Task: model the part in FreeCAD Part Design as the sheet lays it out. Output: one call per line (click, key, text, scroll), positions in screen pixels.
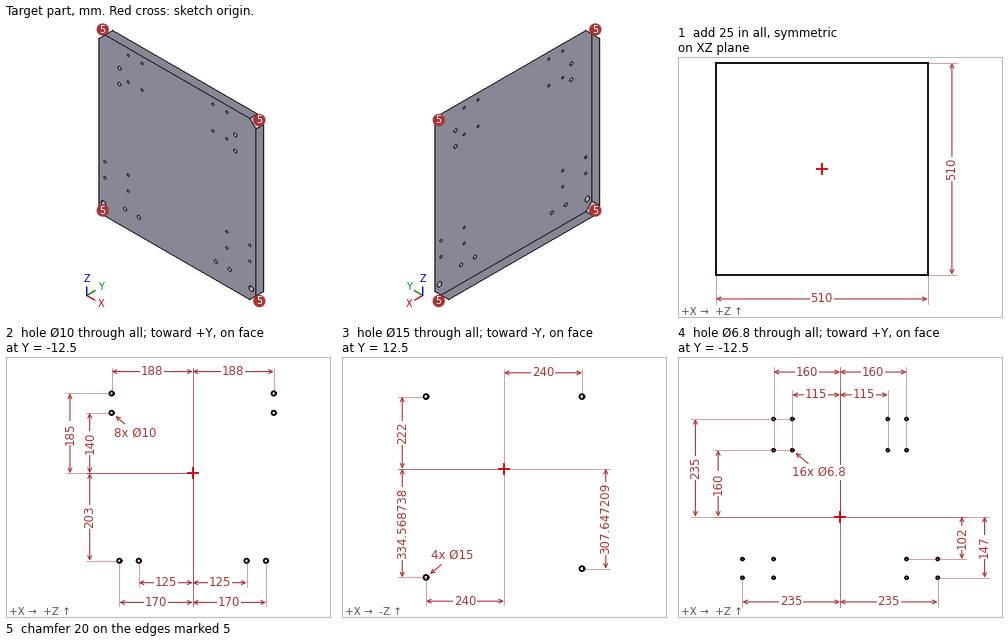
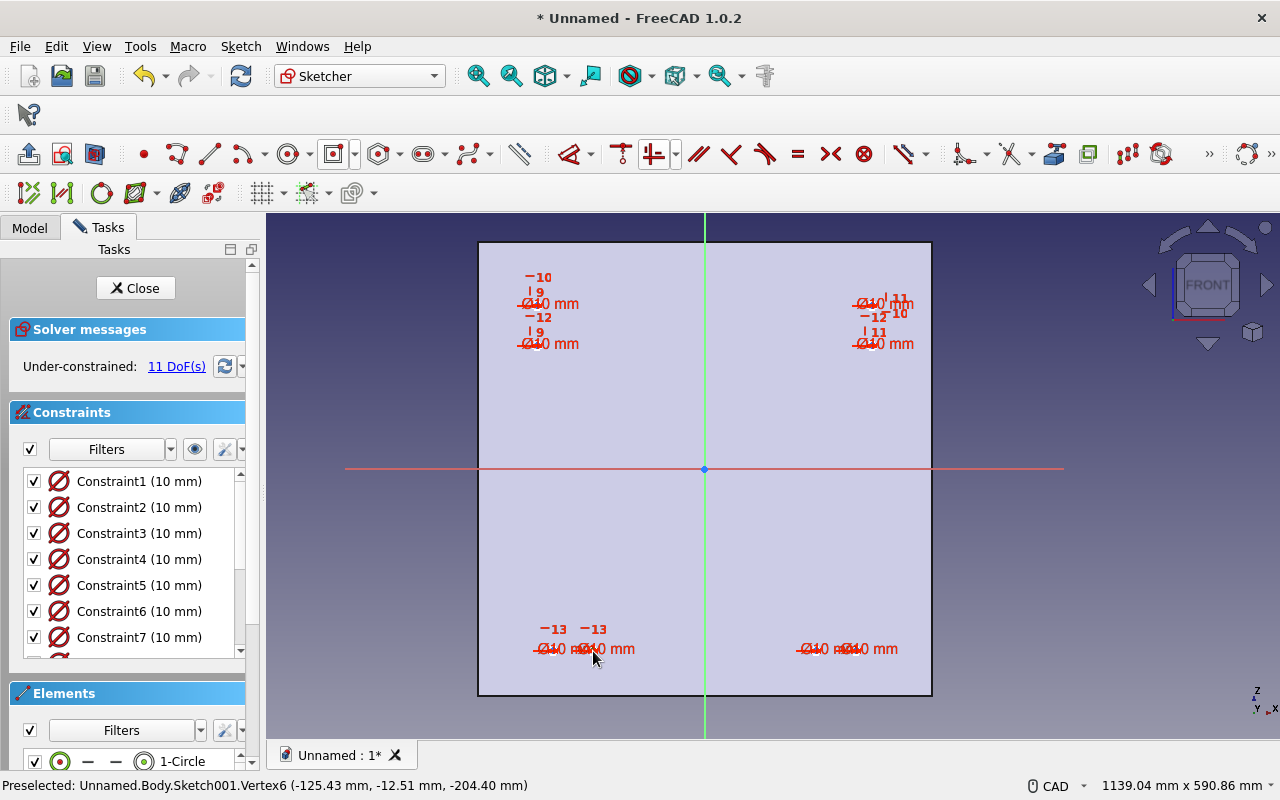
click(816, 651)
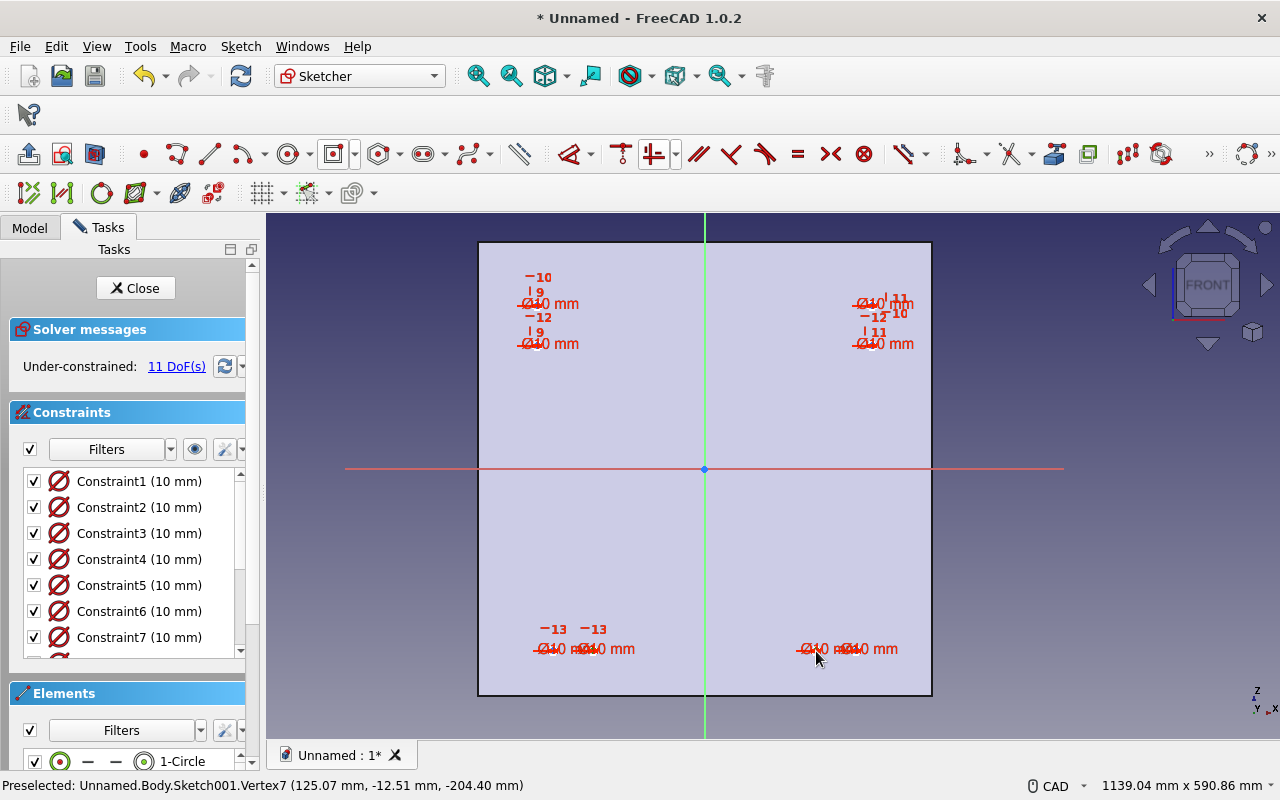
click(676, 154)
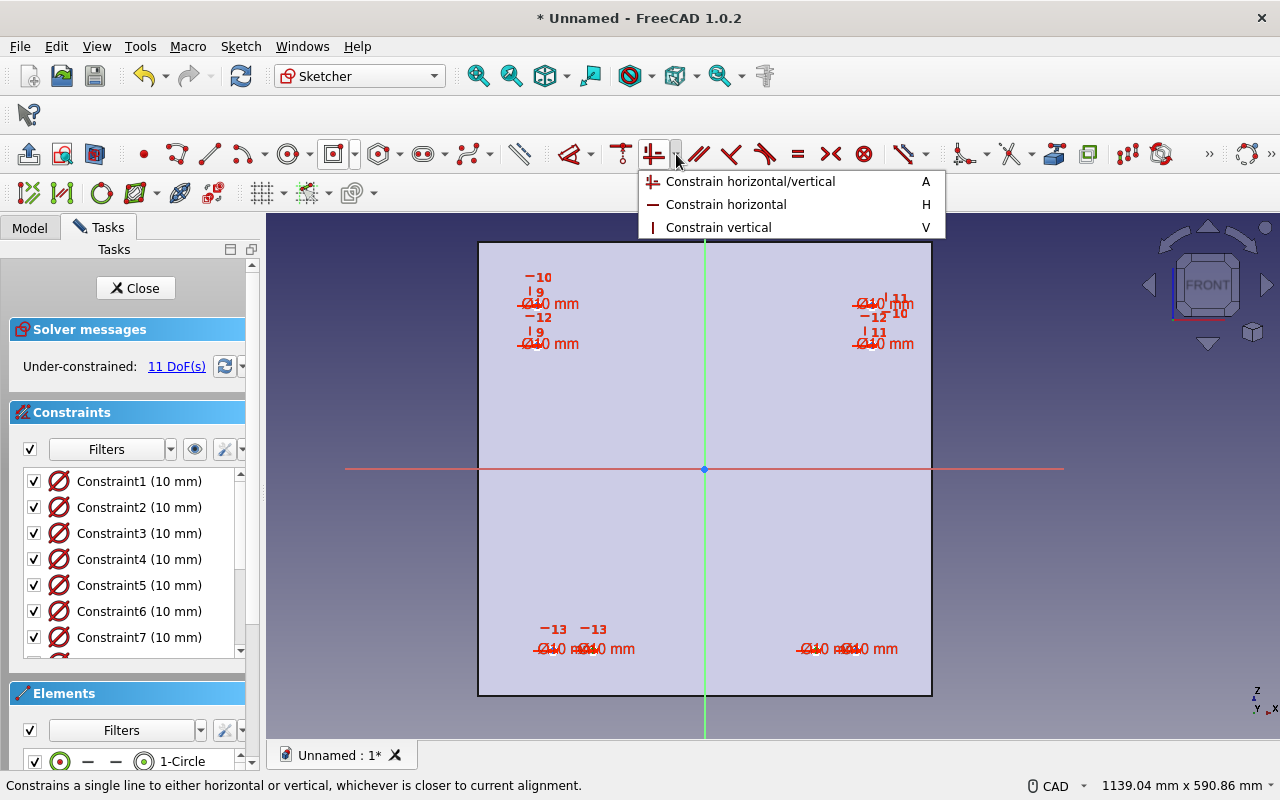
click(792, 204)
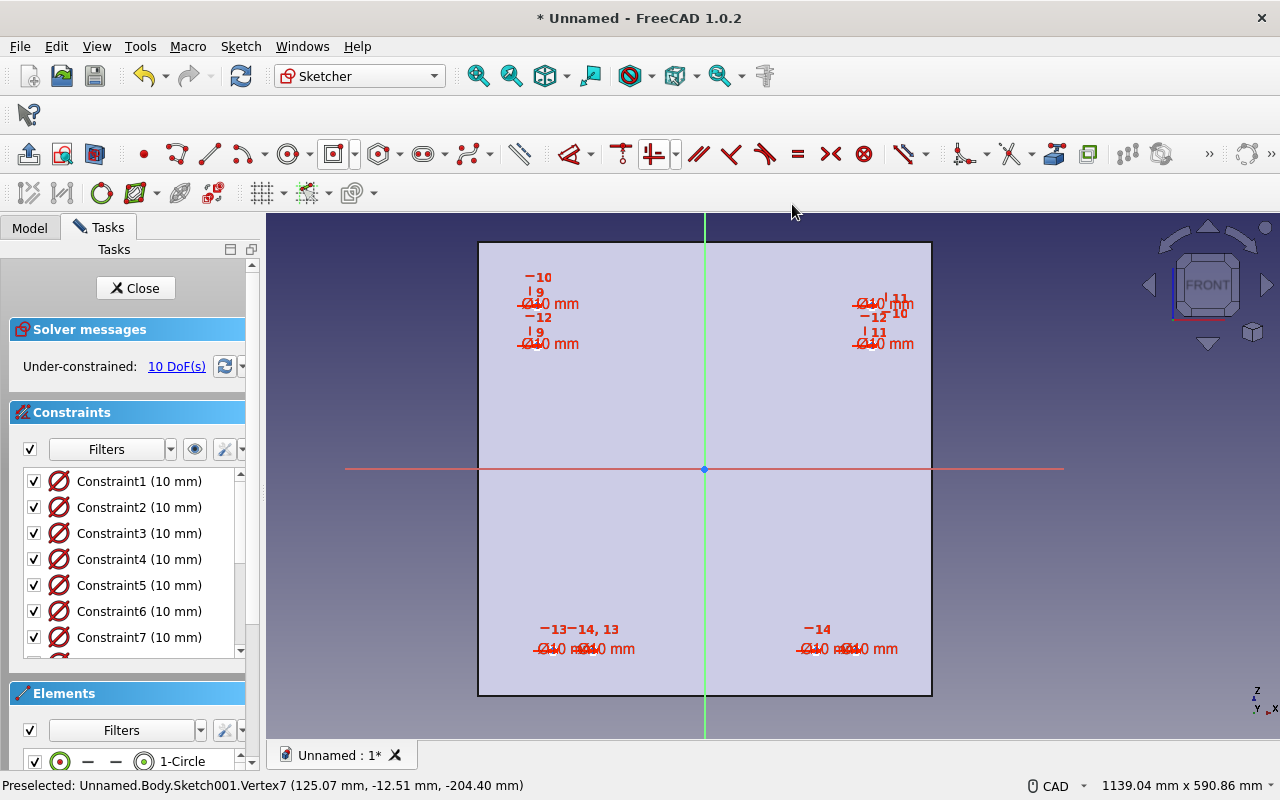
click(816, 651)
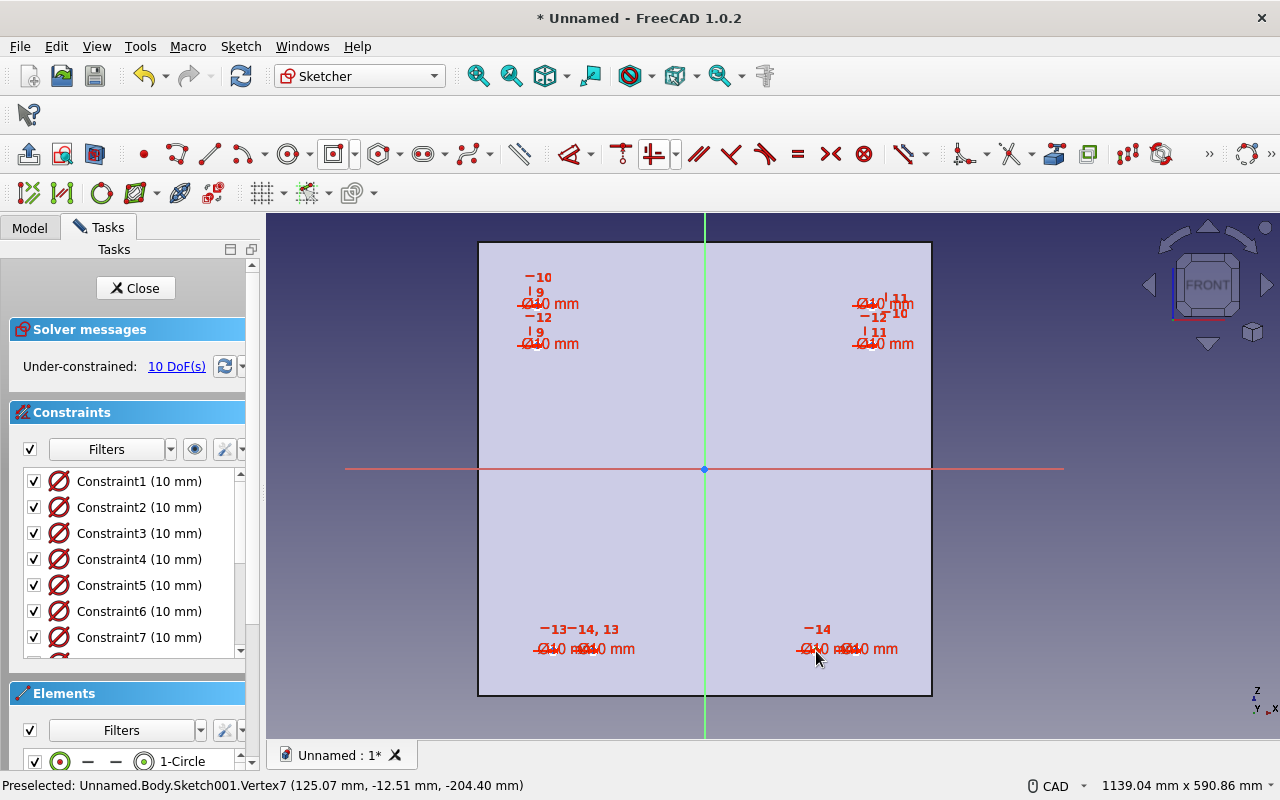
click(856, 651)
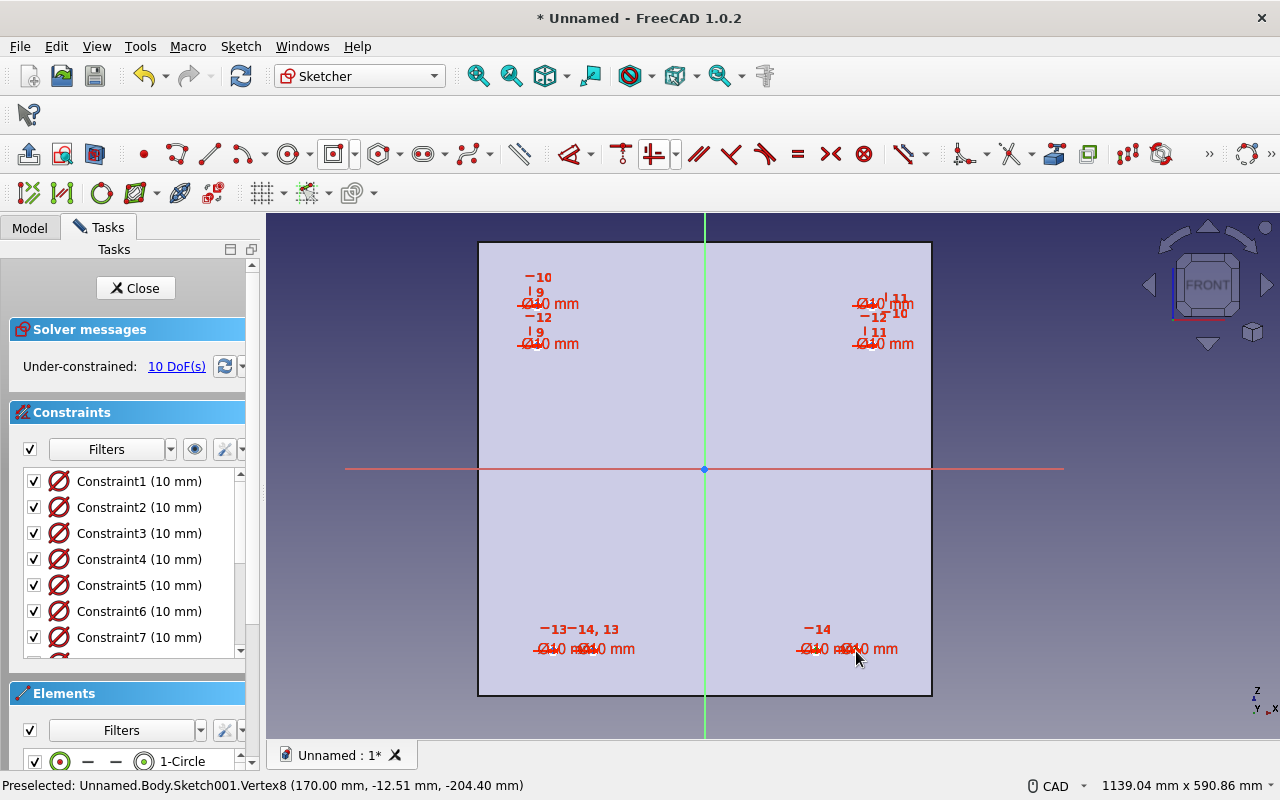
click(676, 154)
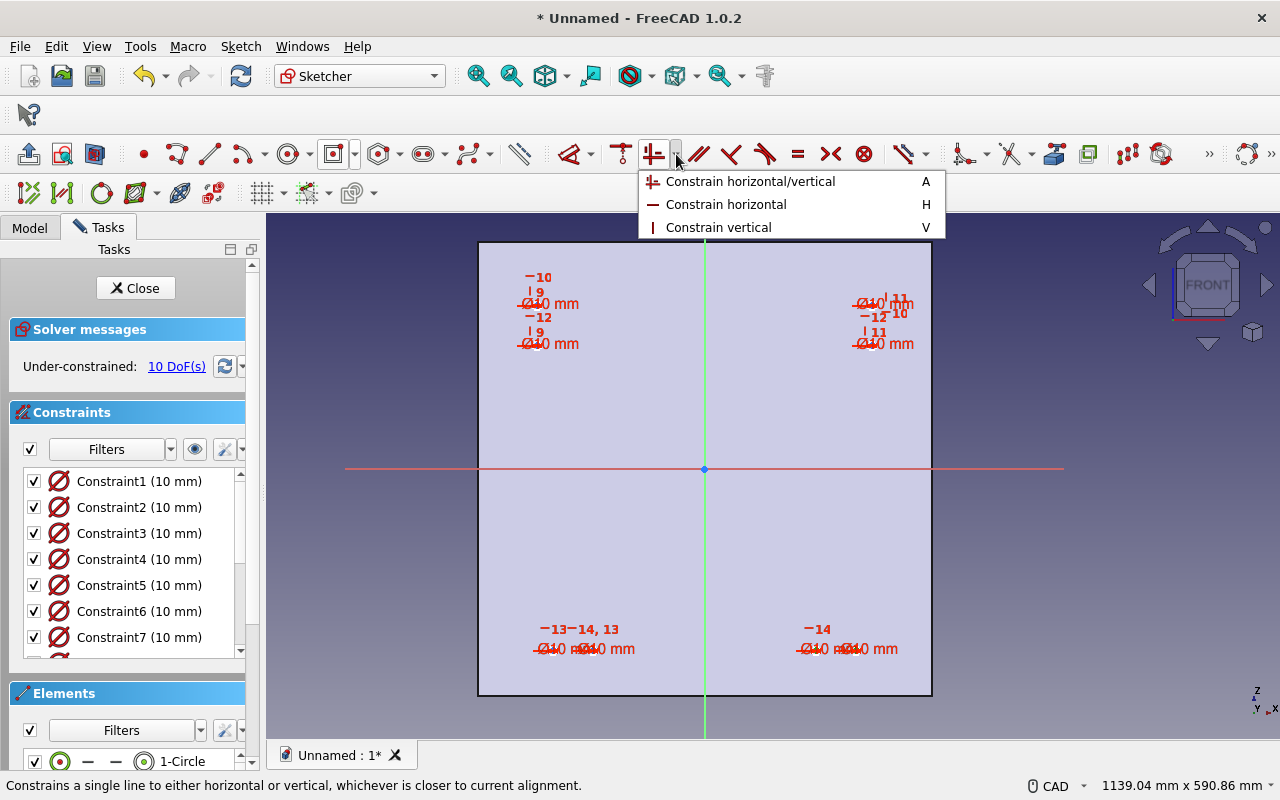
click(792, 204)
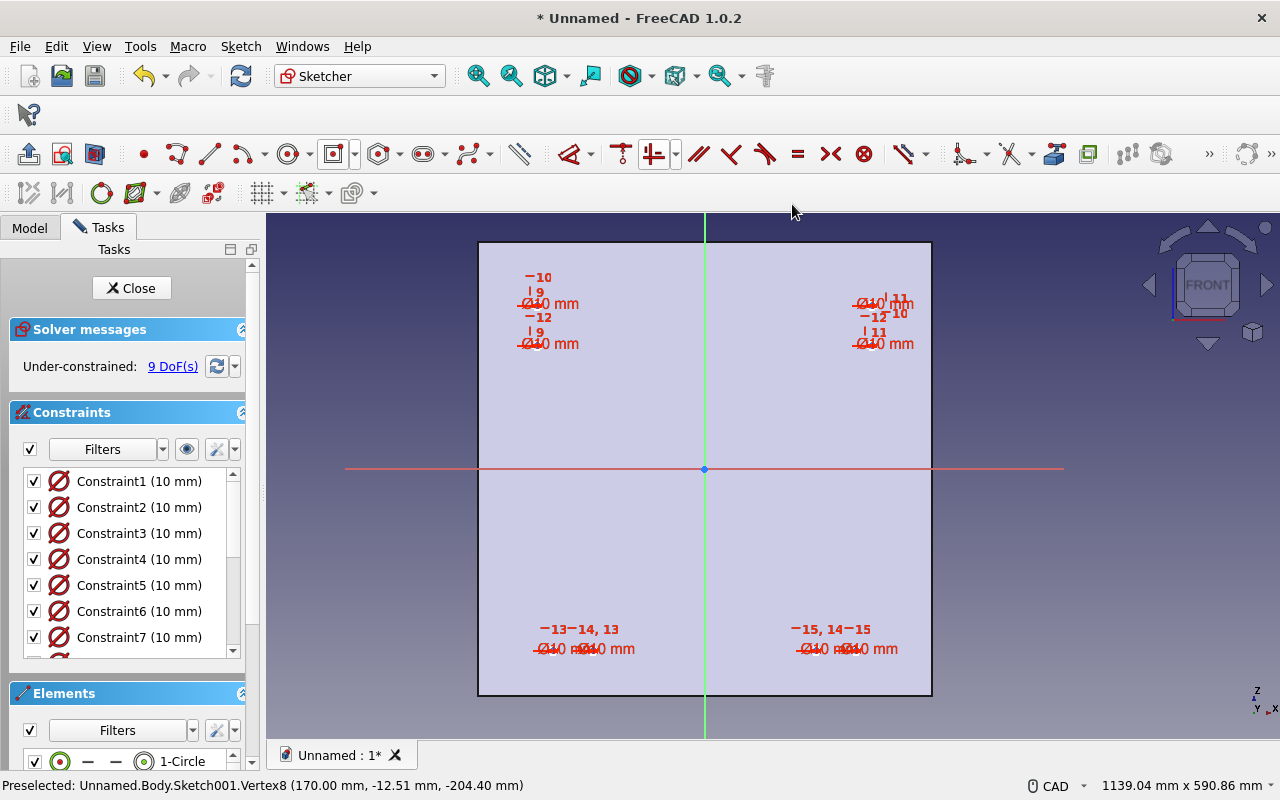
click(537, 306)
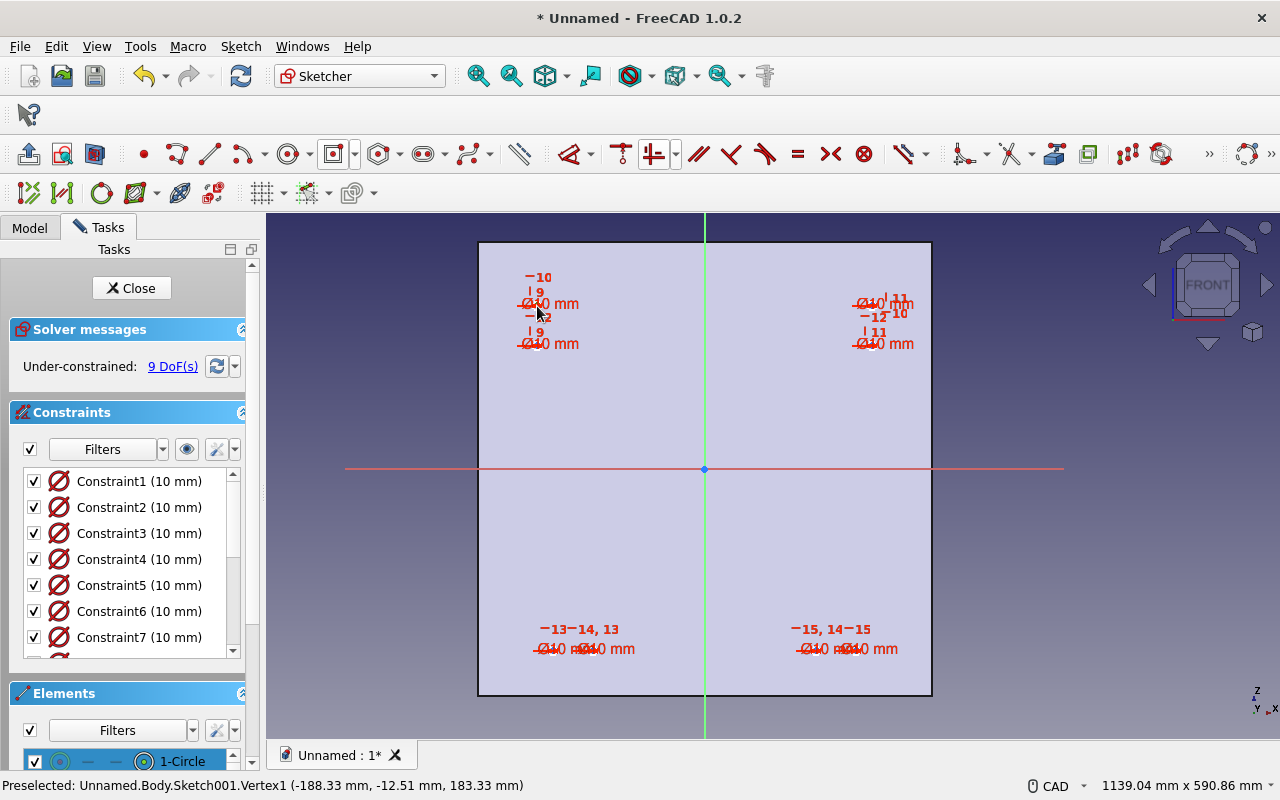
key(l)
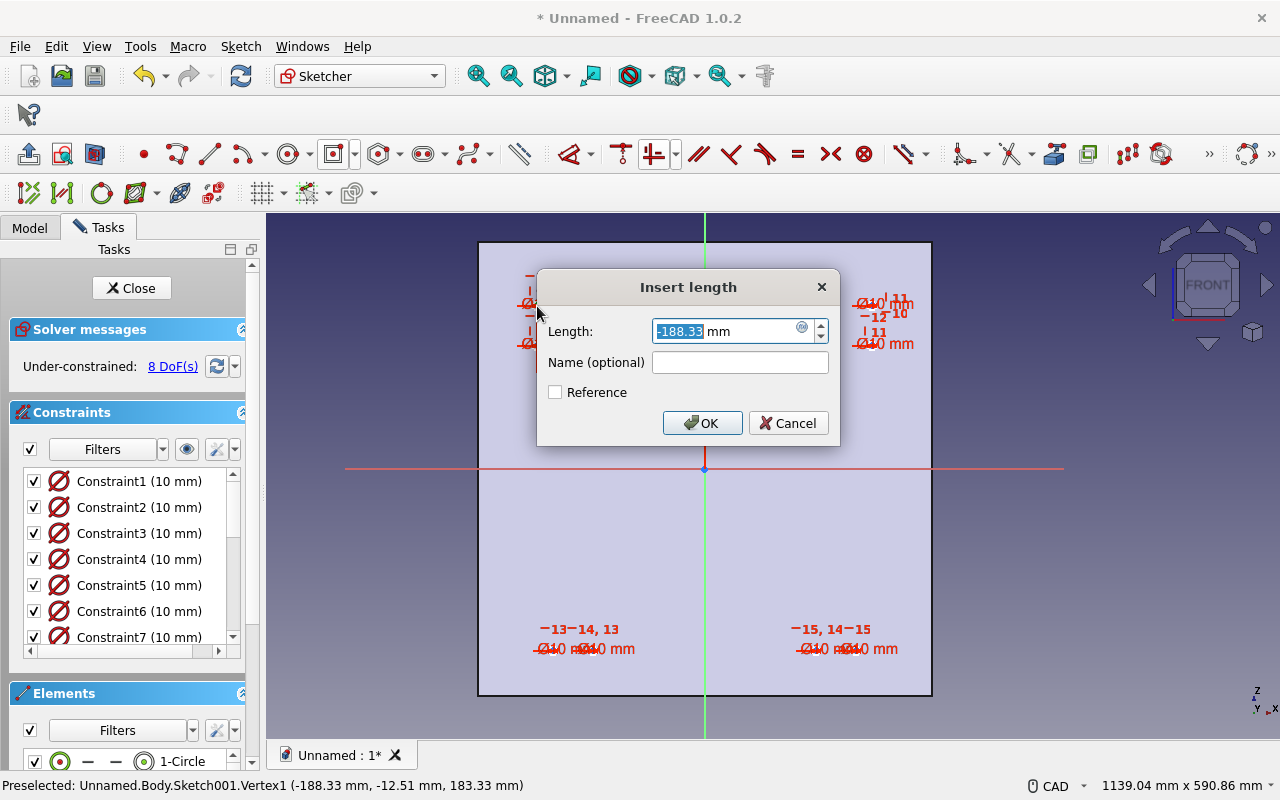
text(-188)
key(Return)